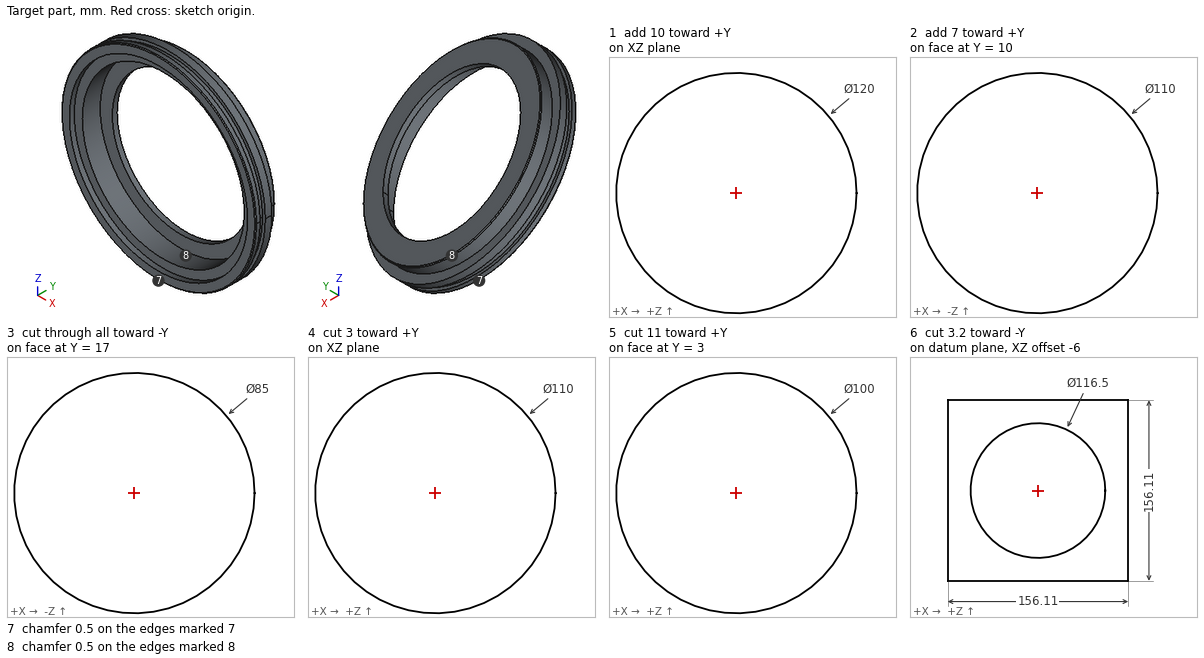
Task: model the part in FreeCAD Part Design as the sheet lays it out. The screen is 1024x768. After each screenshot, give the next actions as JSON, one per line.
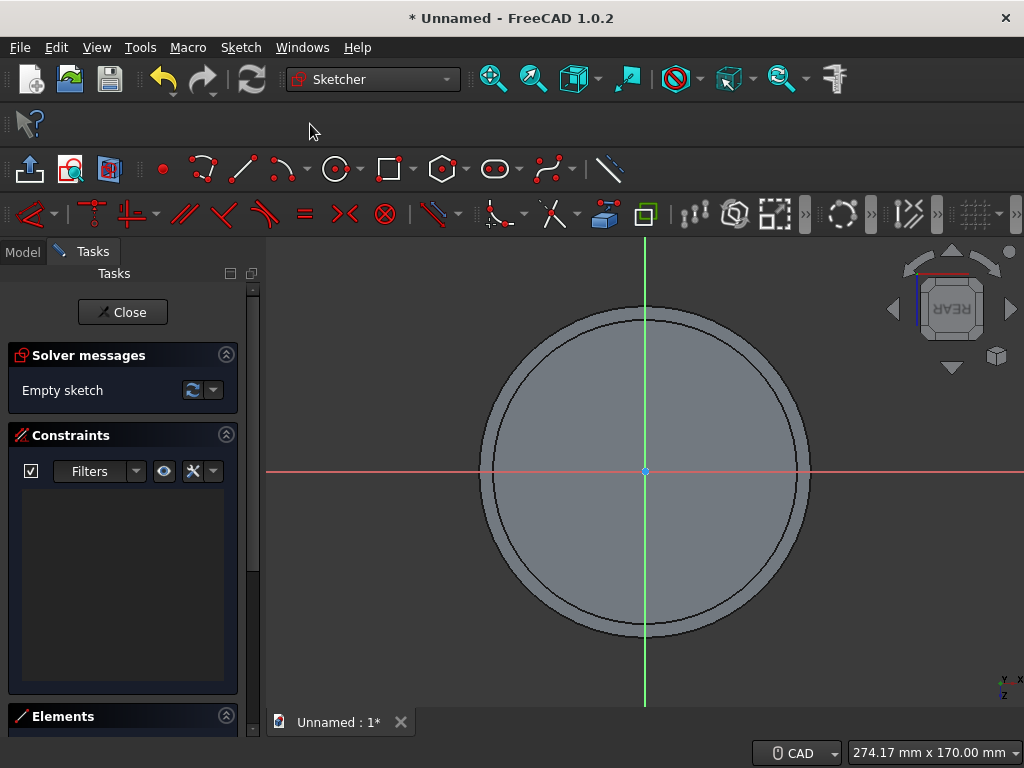
{"action": "left_click", "coordinate": [336, 170]}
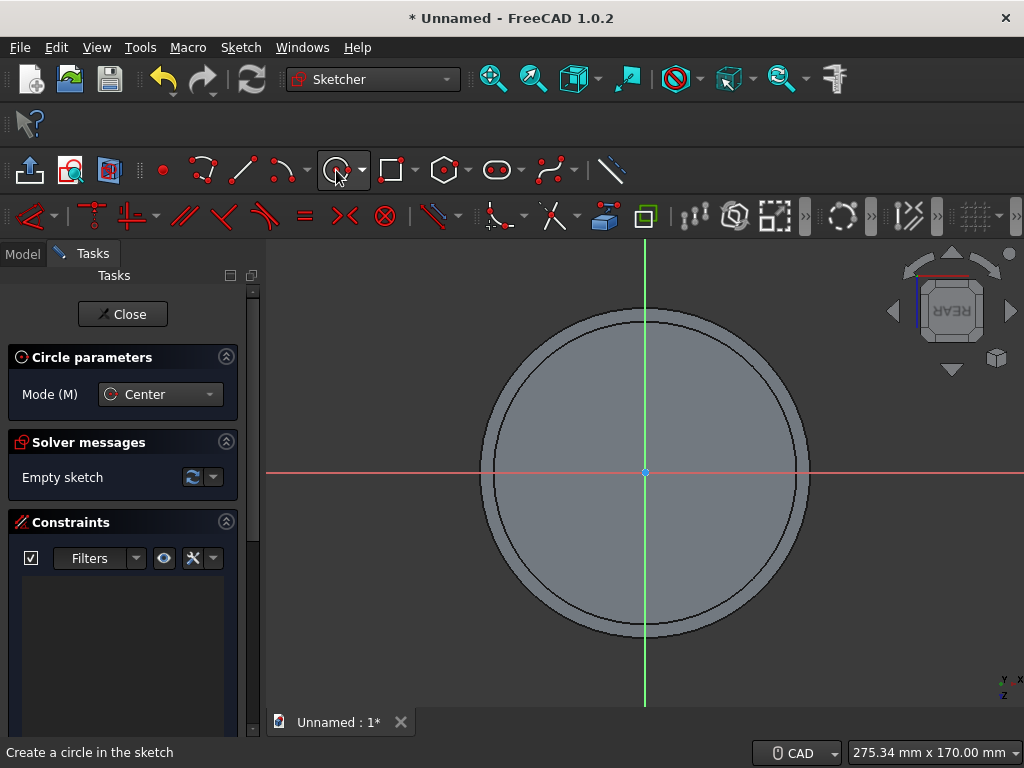
{"action": "left_click", "coordinate": [645, 473]}
{"action": "mouse_move", "coordinate": [728, 390]}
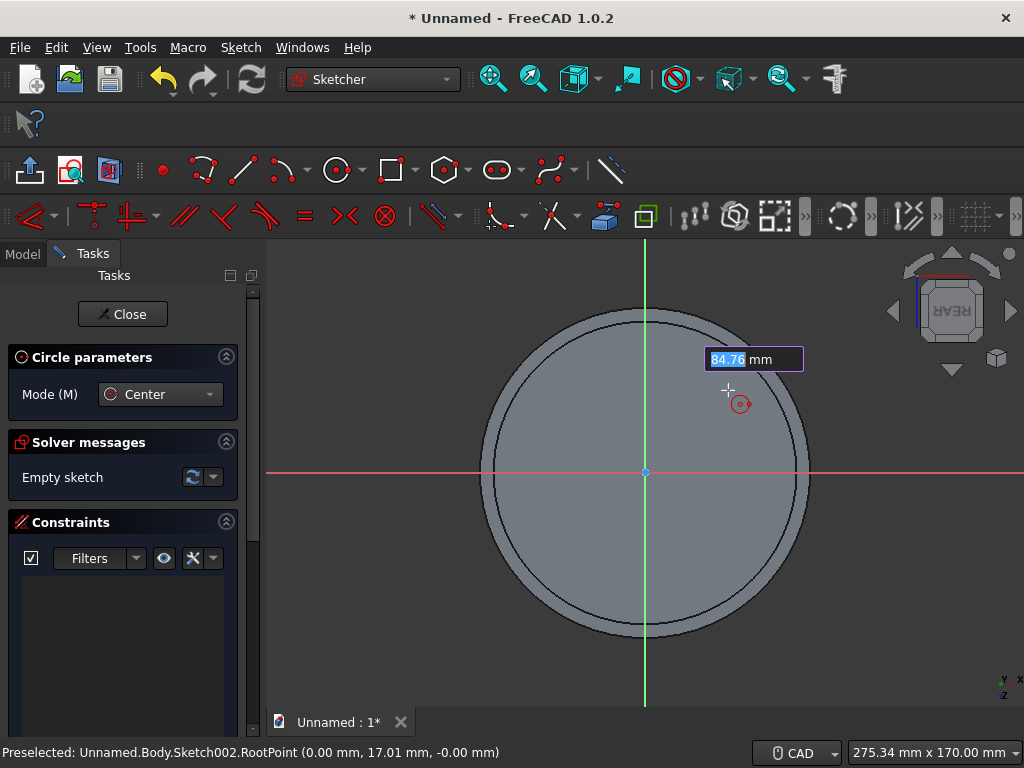
{"action": "type", "text": "85"}
{"action": "key", "text": "Return"}
{"action": "key", "text": "Escape"}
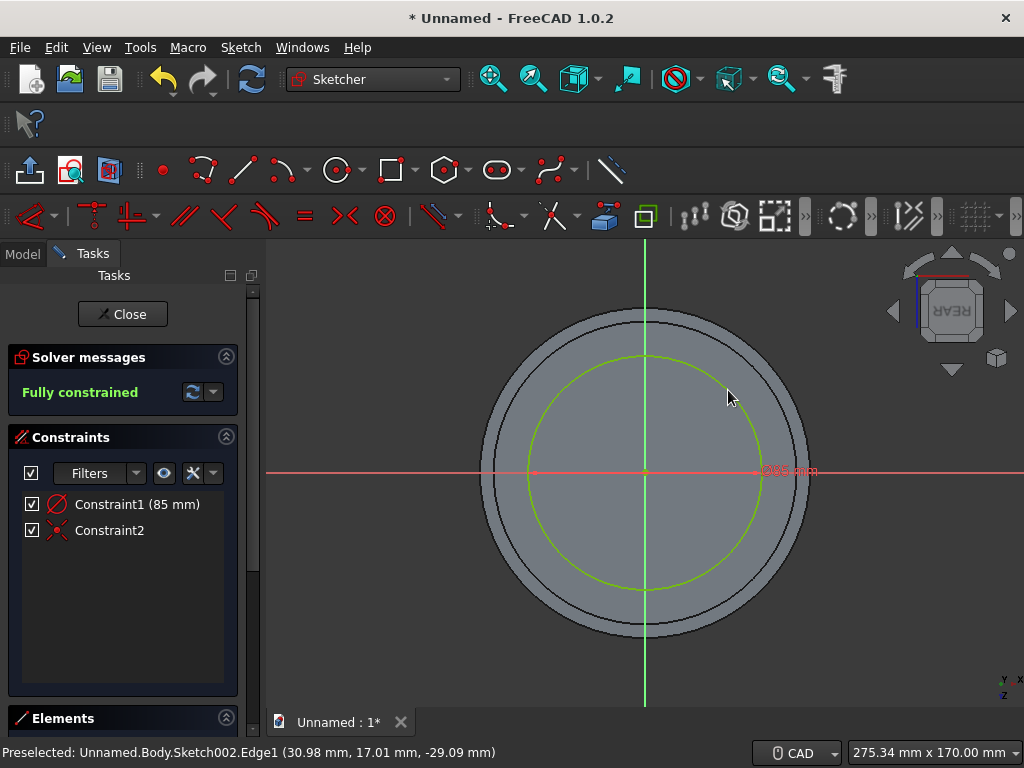
{"action": "left_click", "coordinate": [123, 314]}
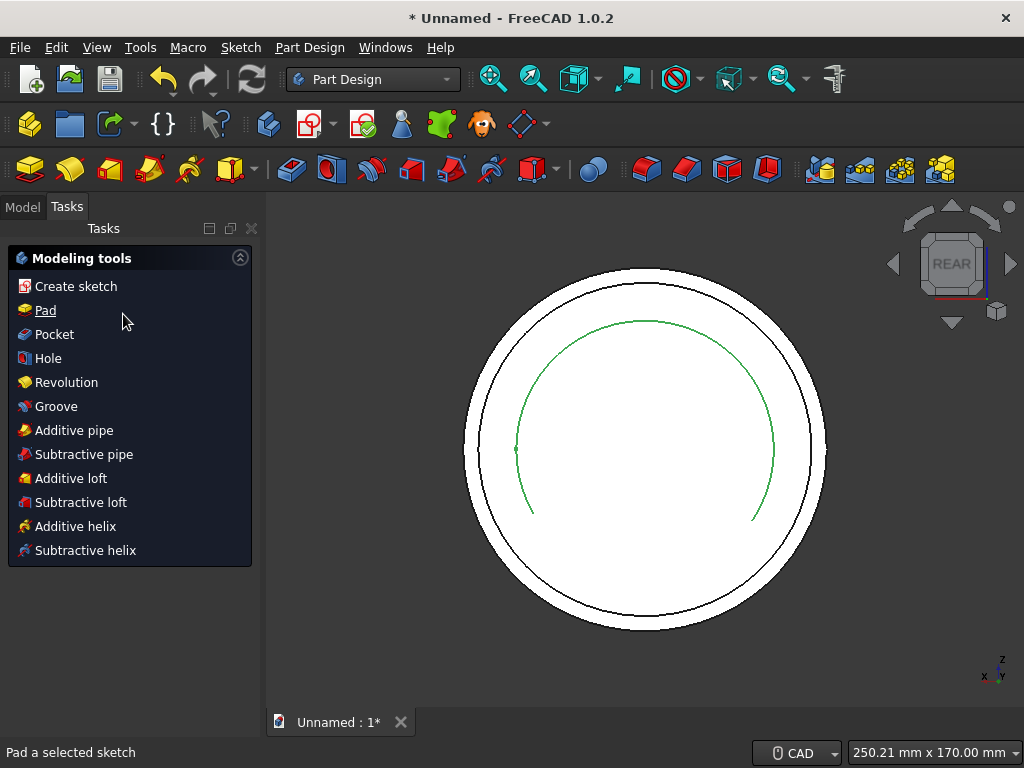
{"action": "left_click", "coordinate": [292, 170]}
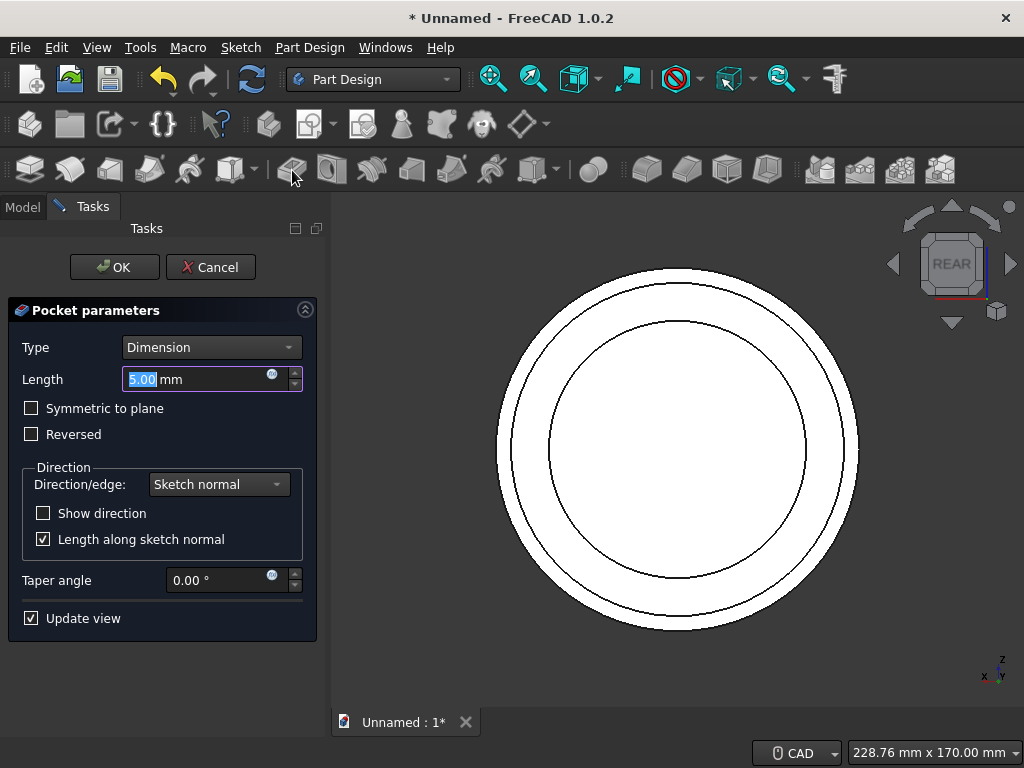
{"action": "left_click", "coordinate": [212, 348]}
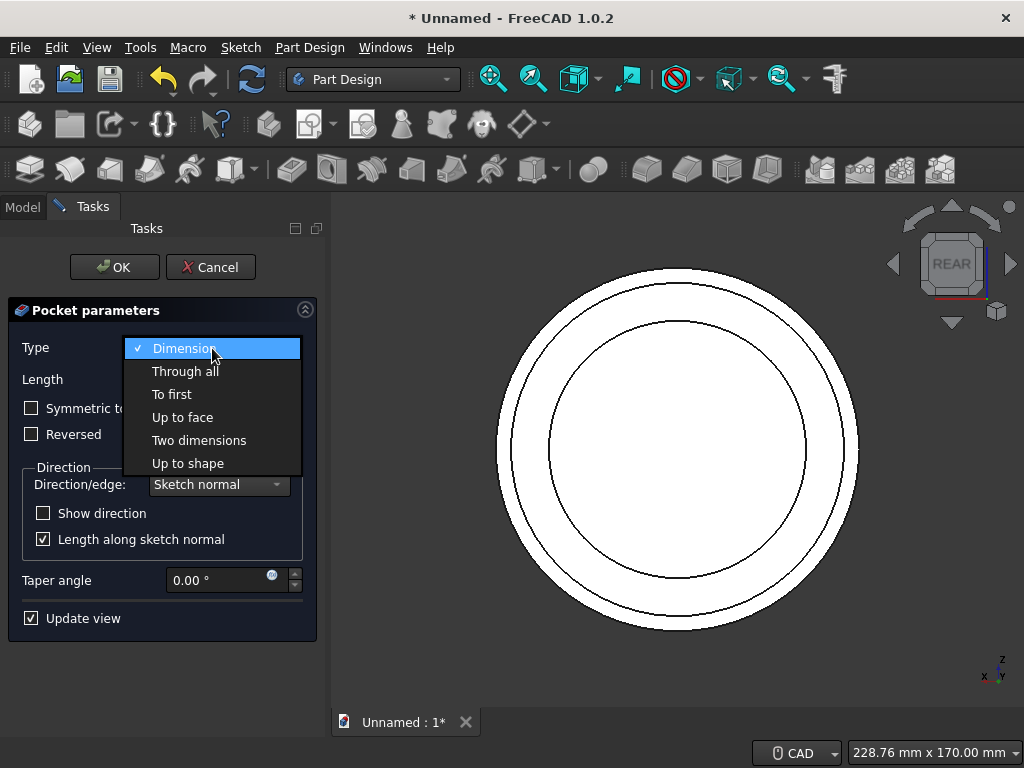
{"action": "left_click", "coordinate": [212, 372]}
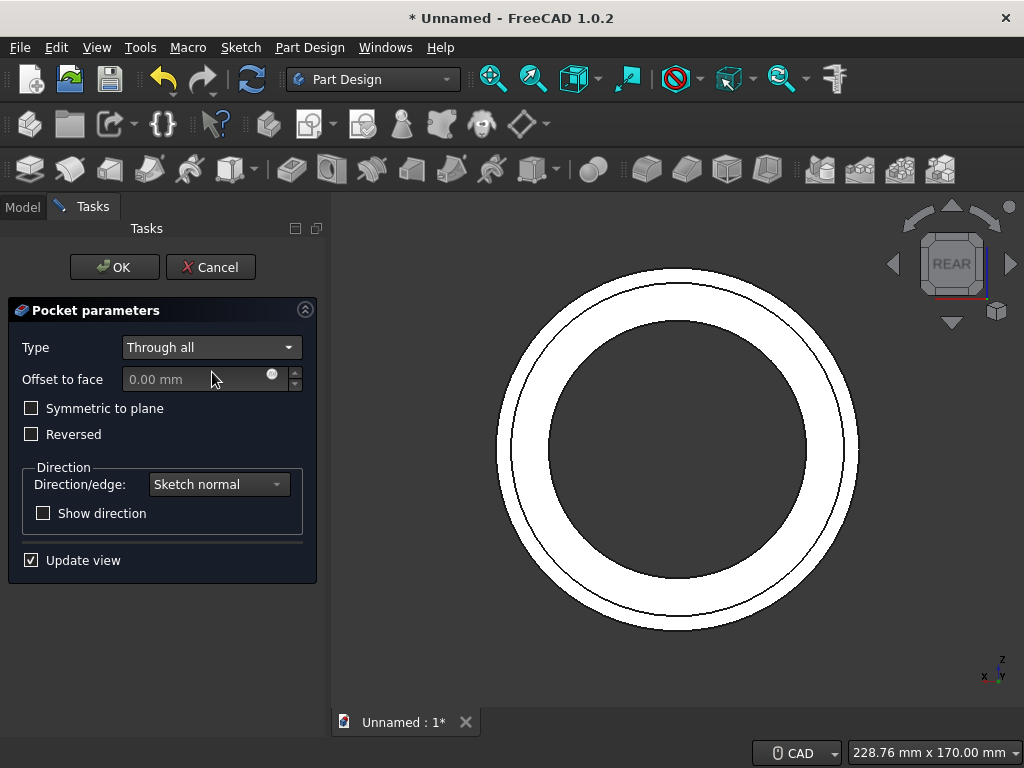
{"action": "left_click", "coordinate": [115, 267]}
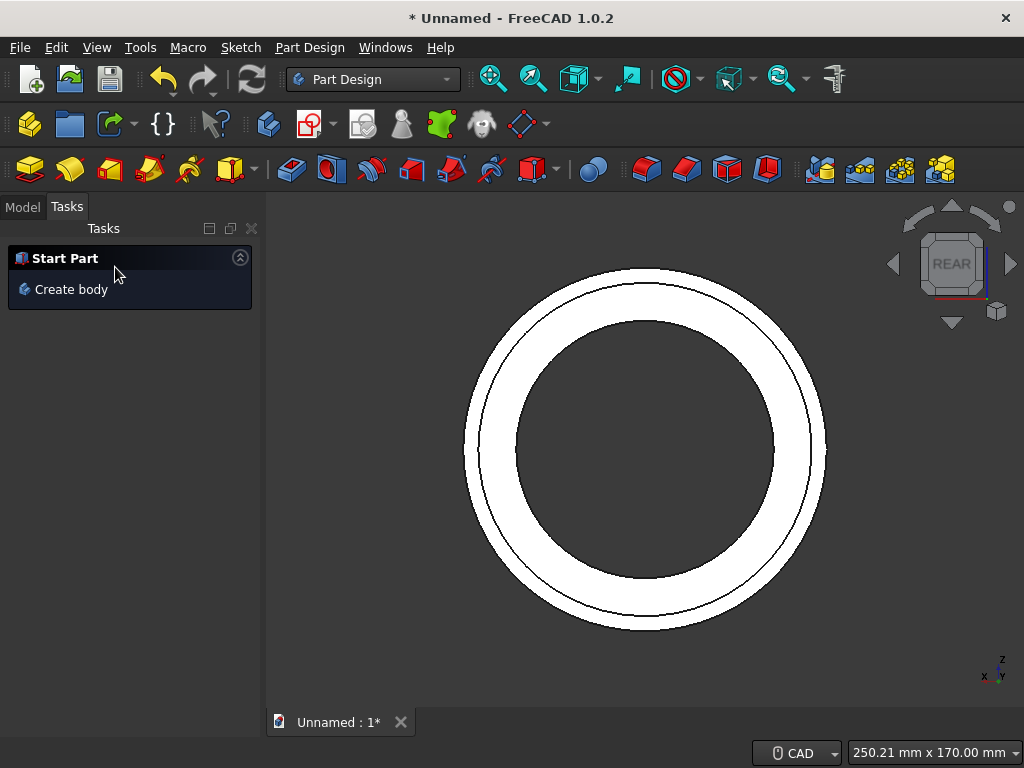
{"action": "left_click", "coordinate": [310, 124]}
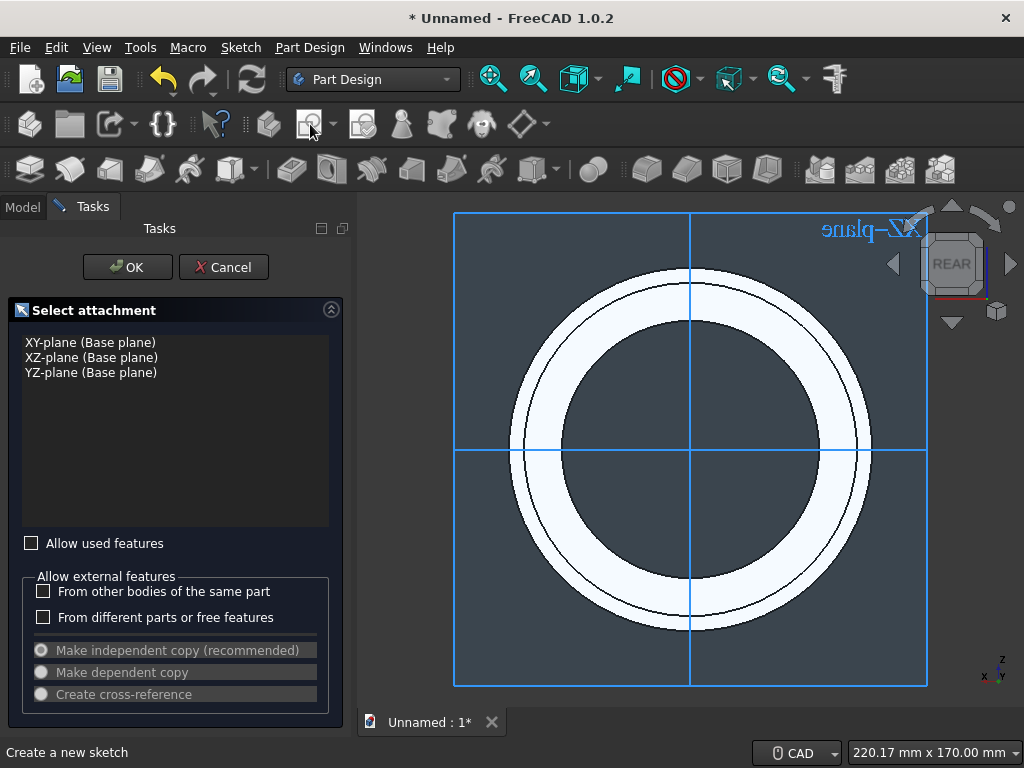
{"action": "left_click", "coordinate": [82, 358]}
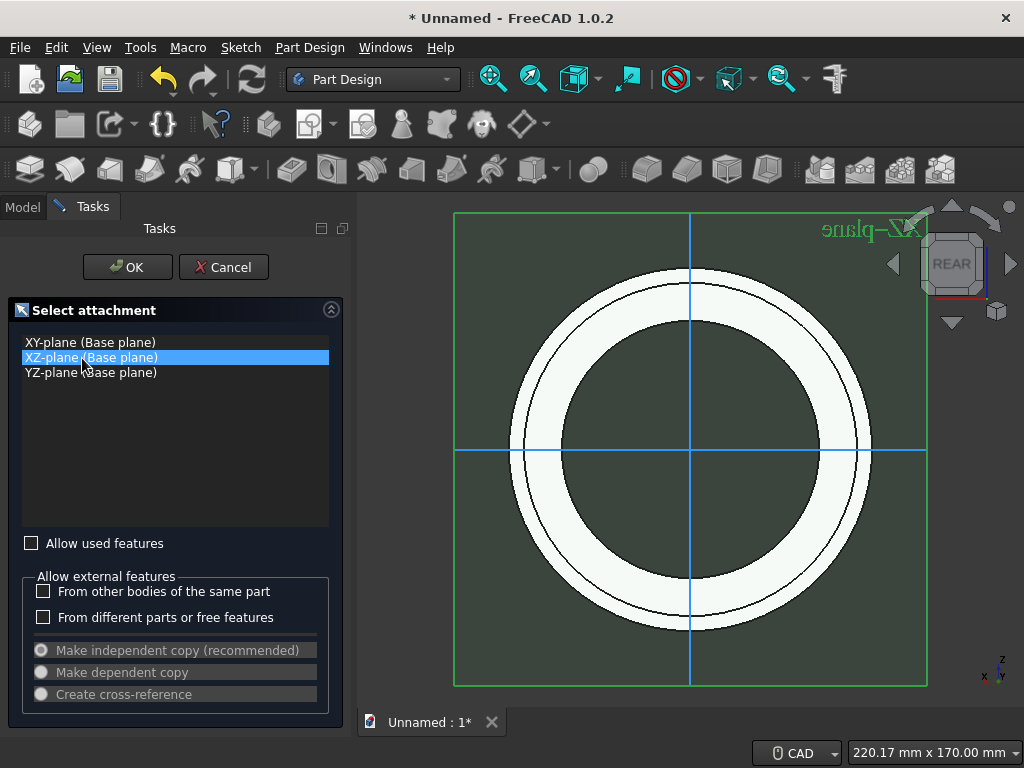
{"action": "left_click", "coordinate": [128, 267]}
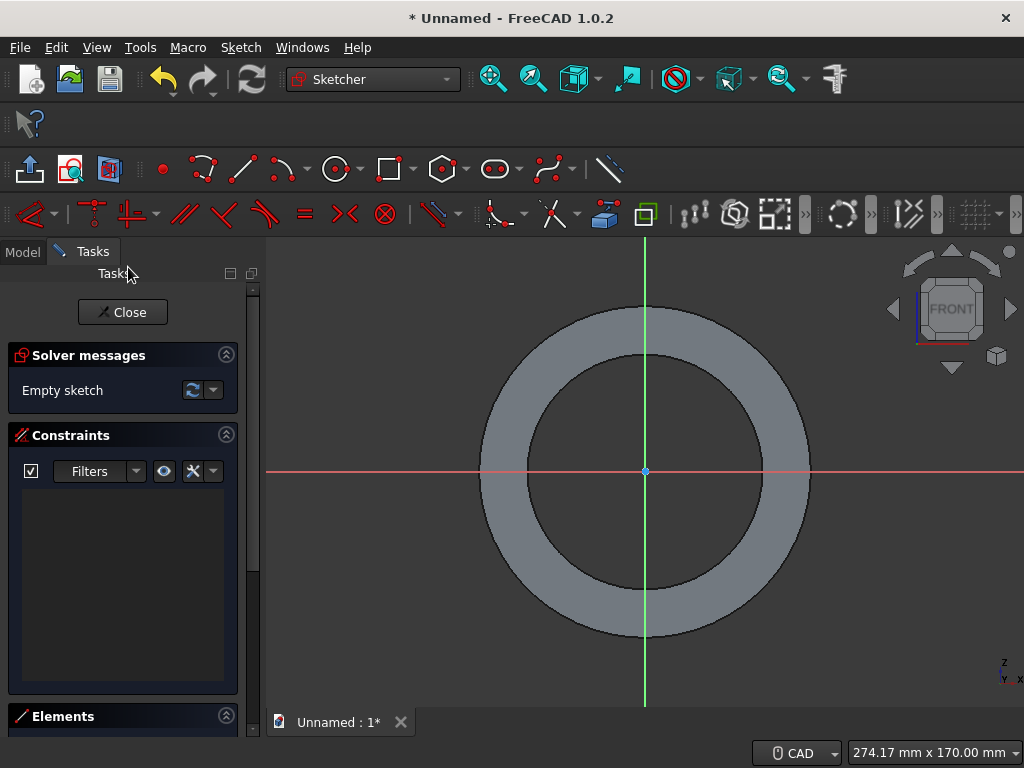
{"action": "left_click", "coordinate": [336, 170]}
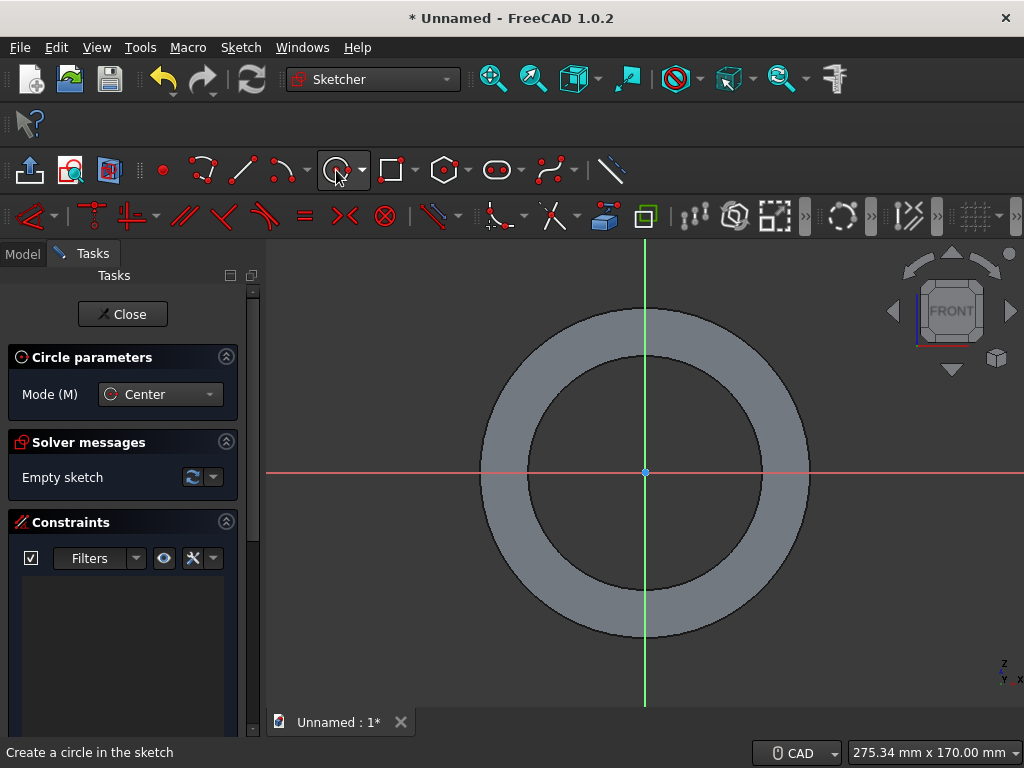
{"action": "left_click", "coordinate": [645, 473]}
{"action": "mouse_move", "coordinate": [752, 366]}